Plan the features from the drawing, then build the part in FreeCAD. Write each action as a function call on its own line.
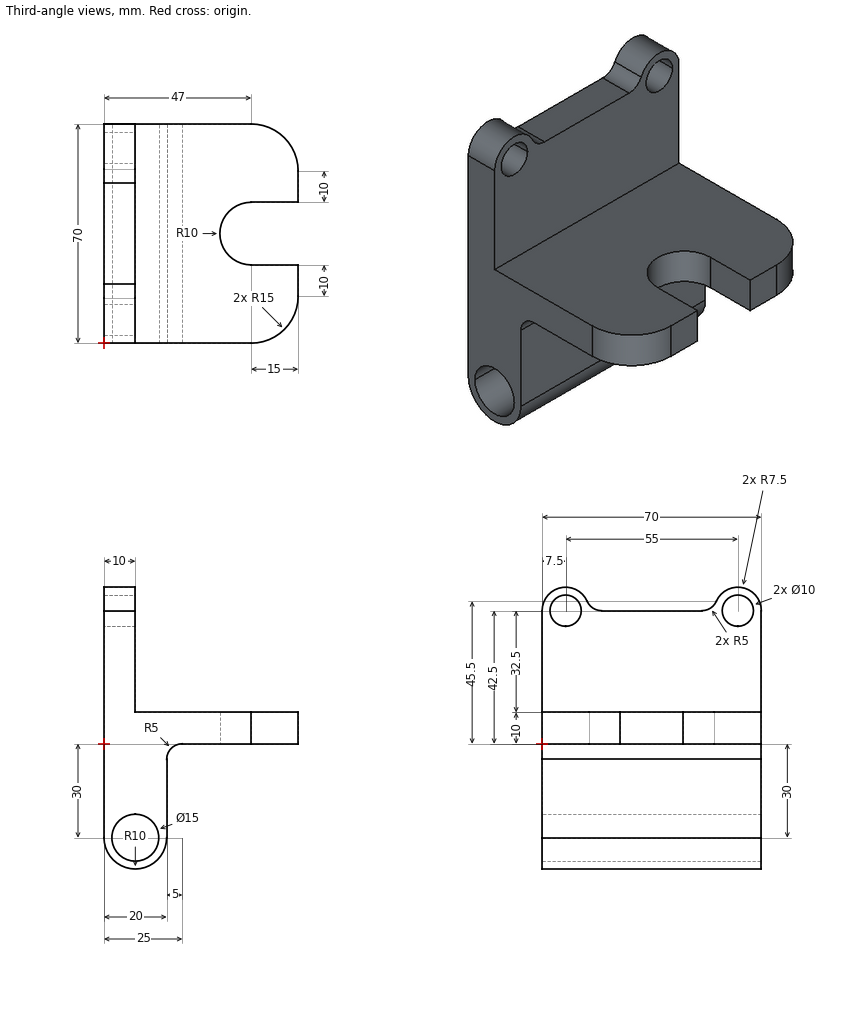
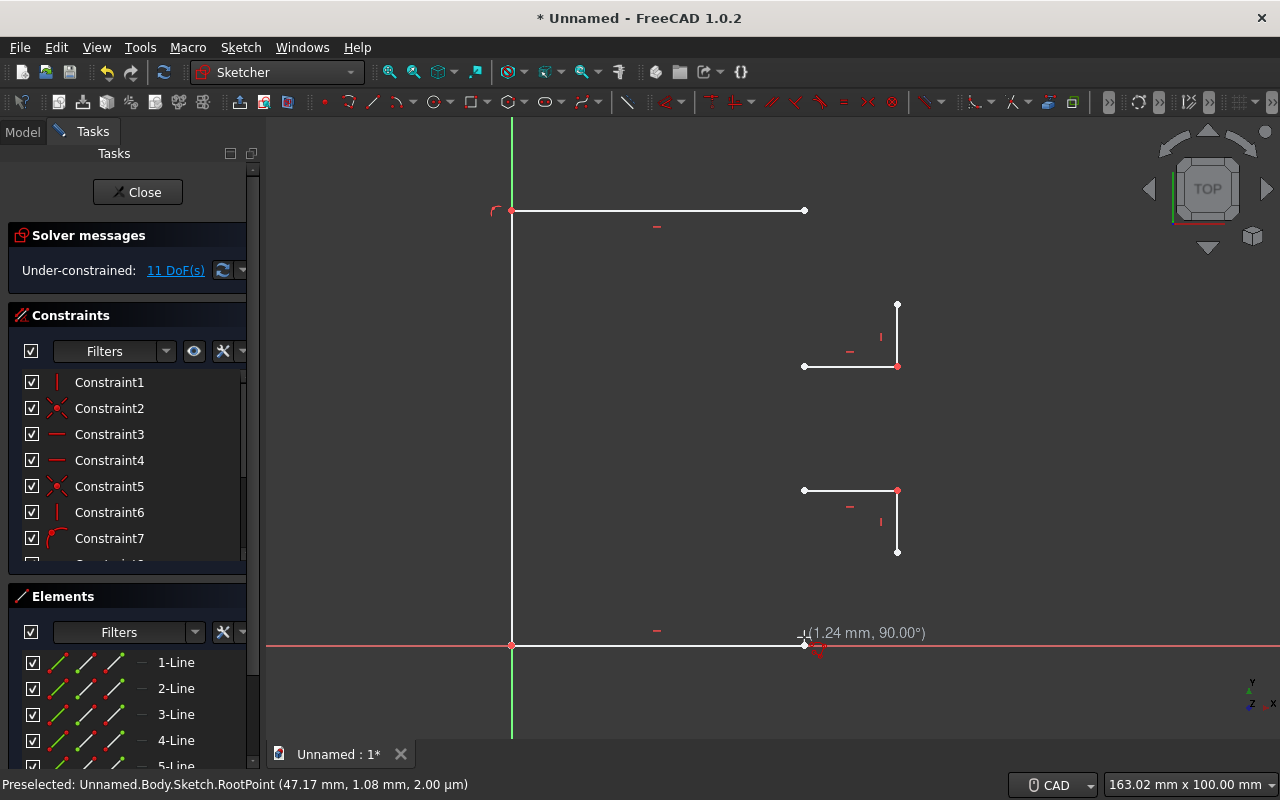
key(g)
key(3)
key(a)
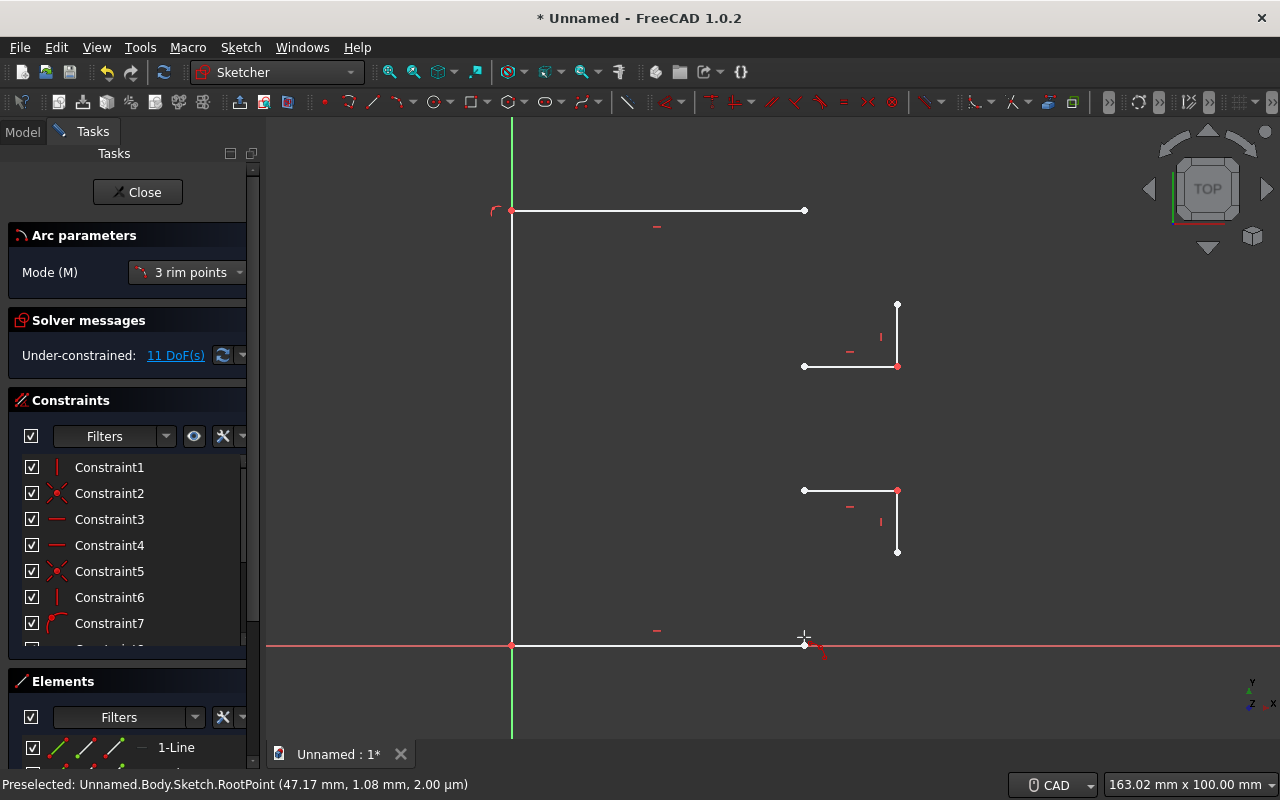
click(804, 491)
click(804, 367)
click(742, 428)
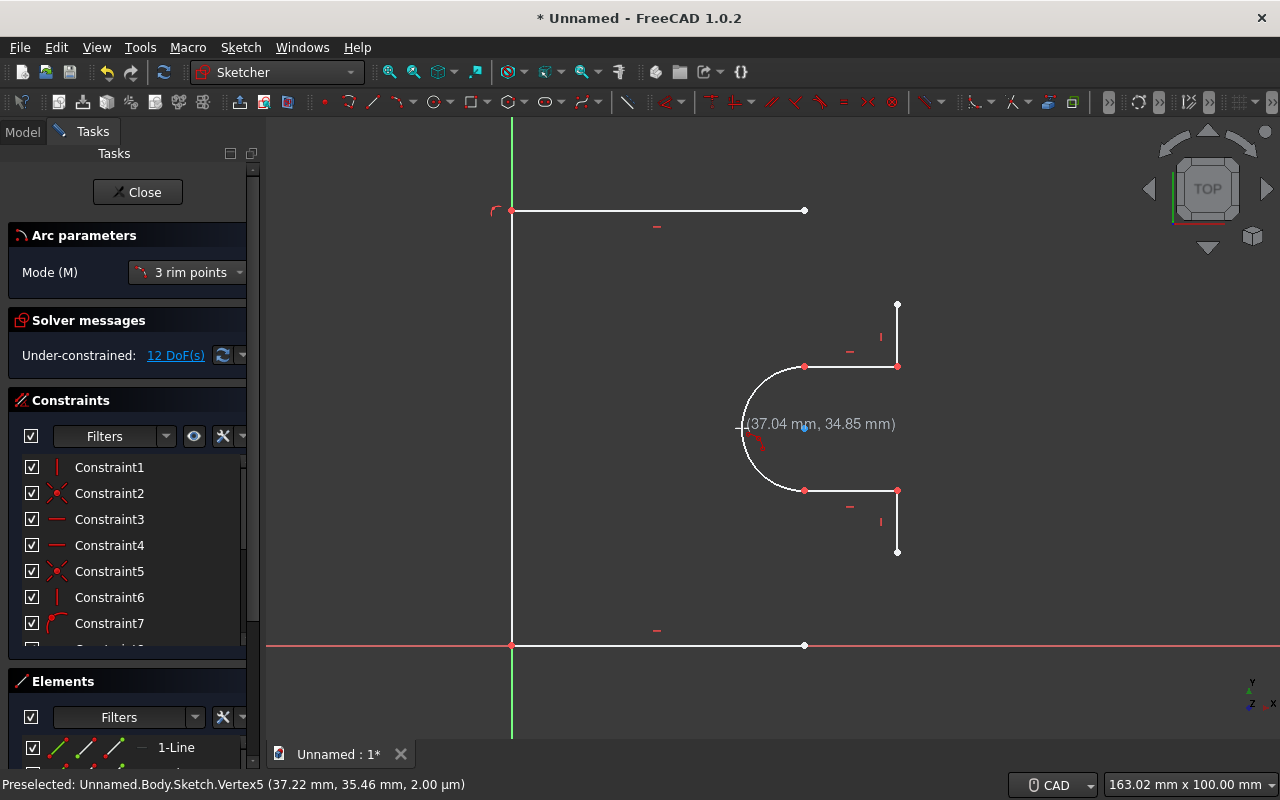
click(897, 305)
click(804, 211)
click(870, 238)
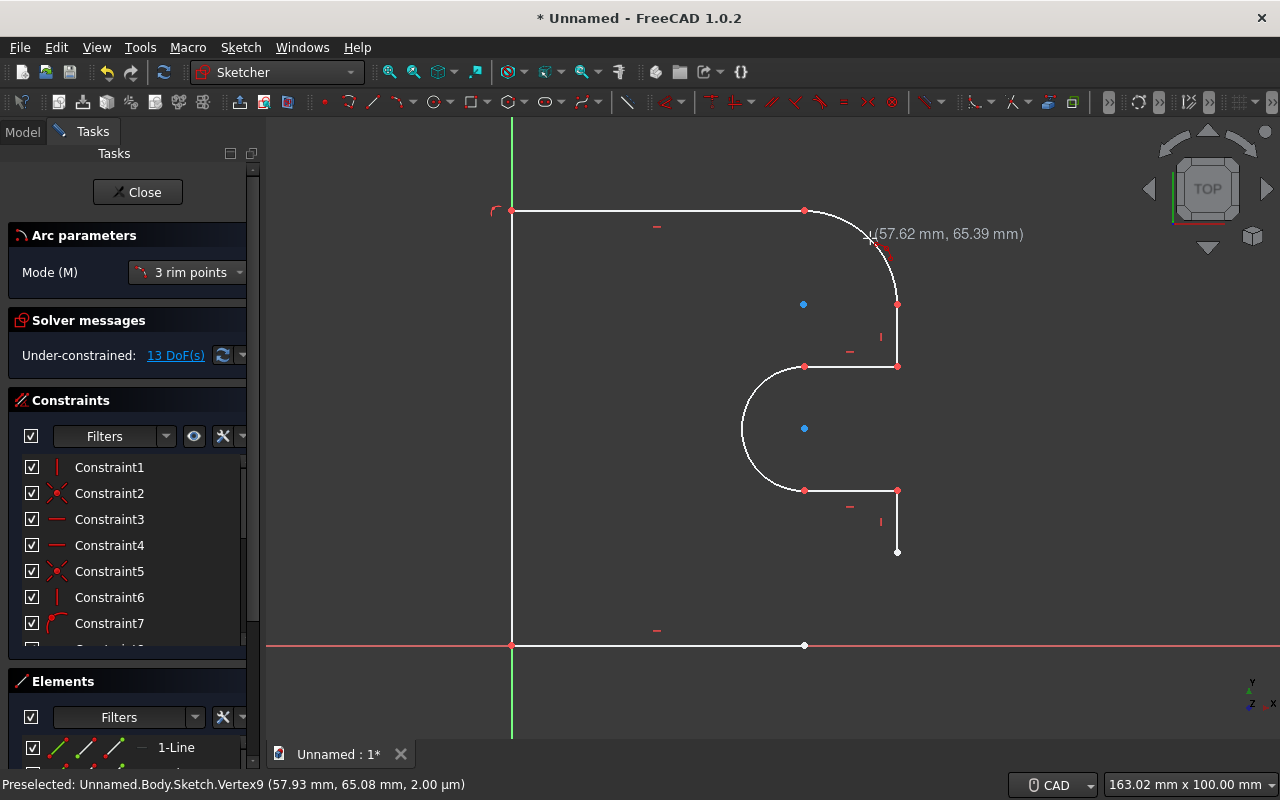
click(804, 646)
click(897, 553)
click(870, 618)
key(Escape)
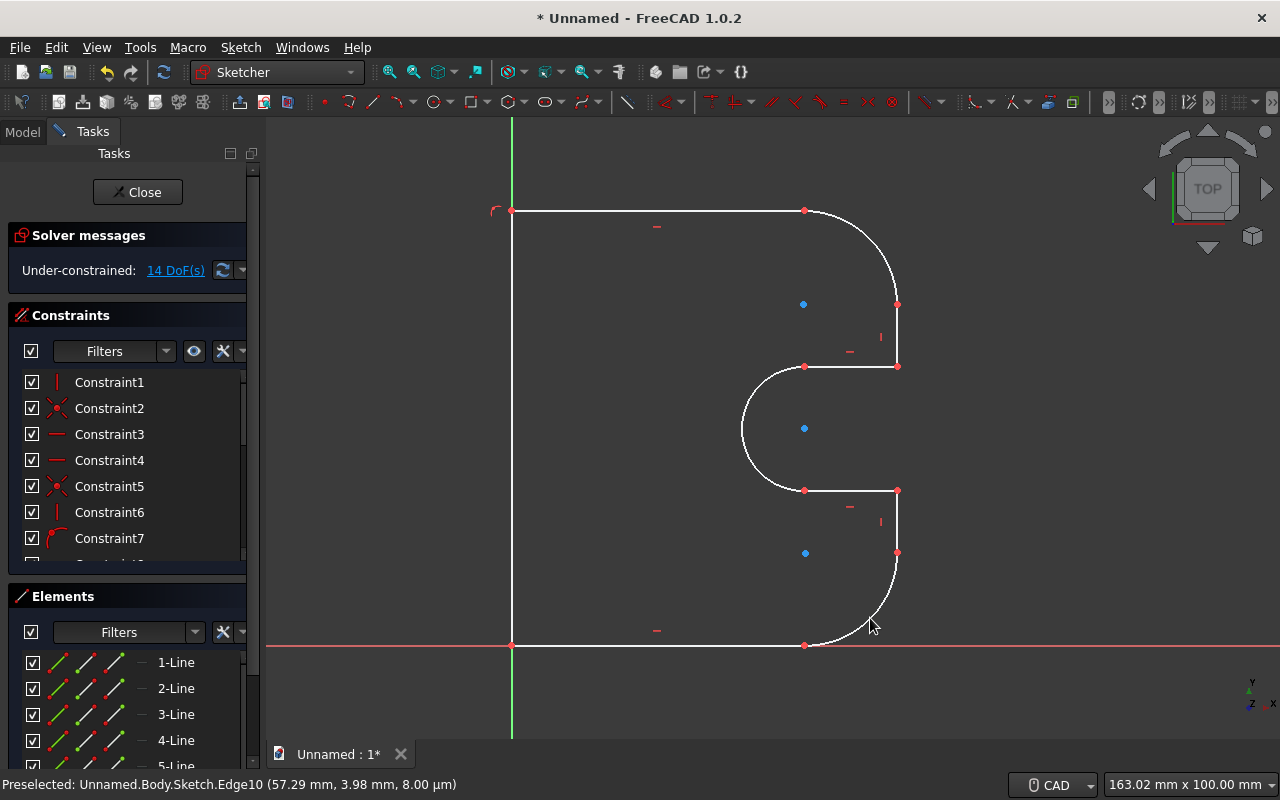
click(897, 534)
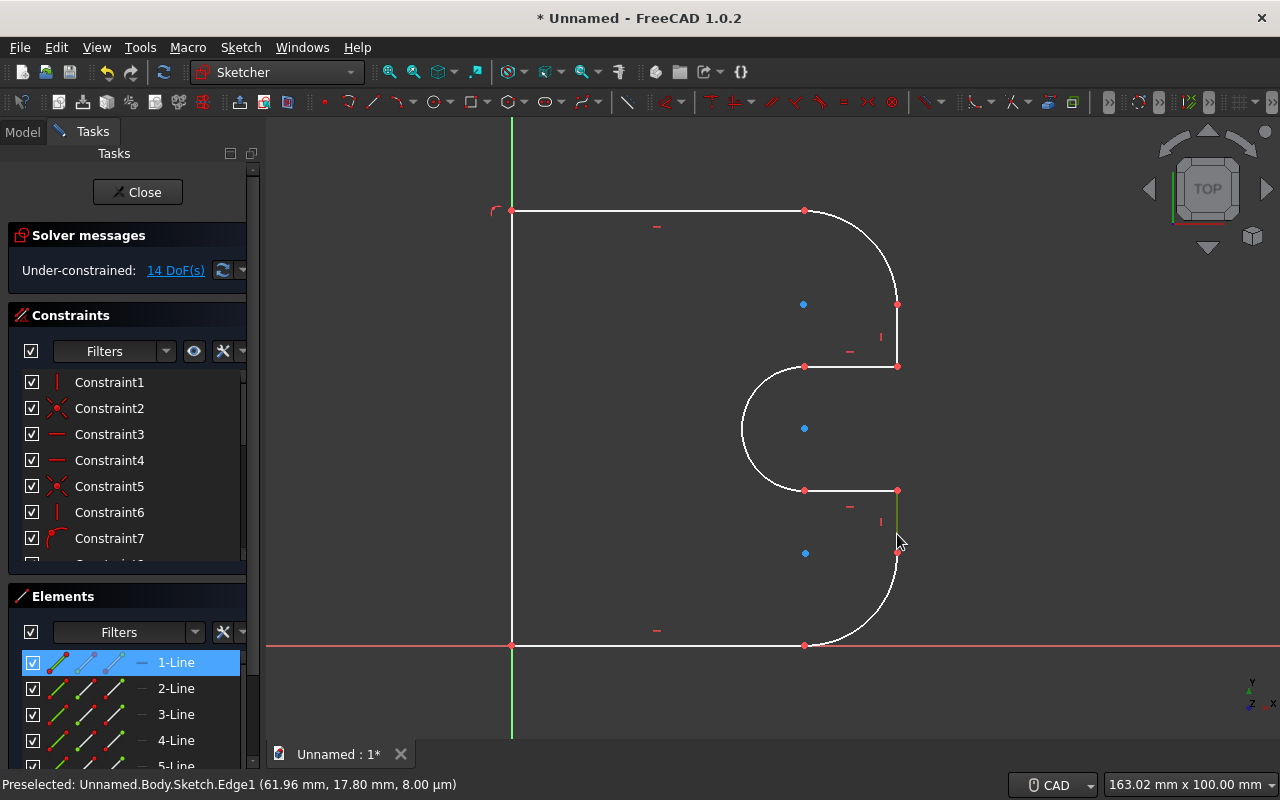
scroll(846, 636, up, 2)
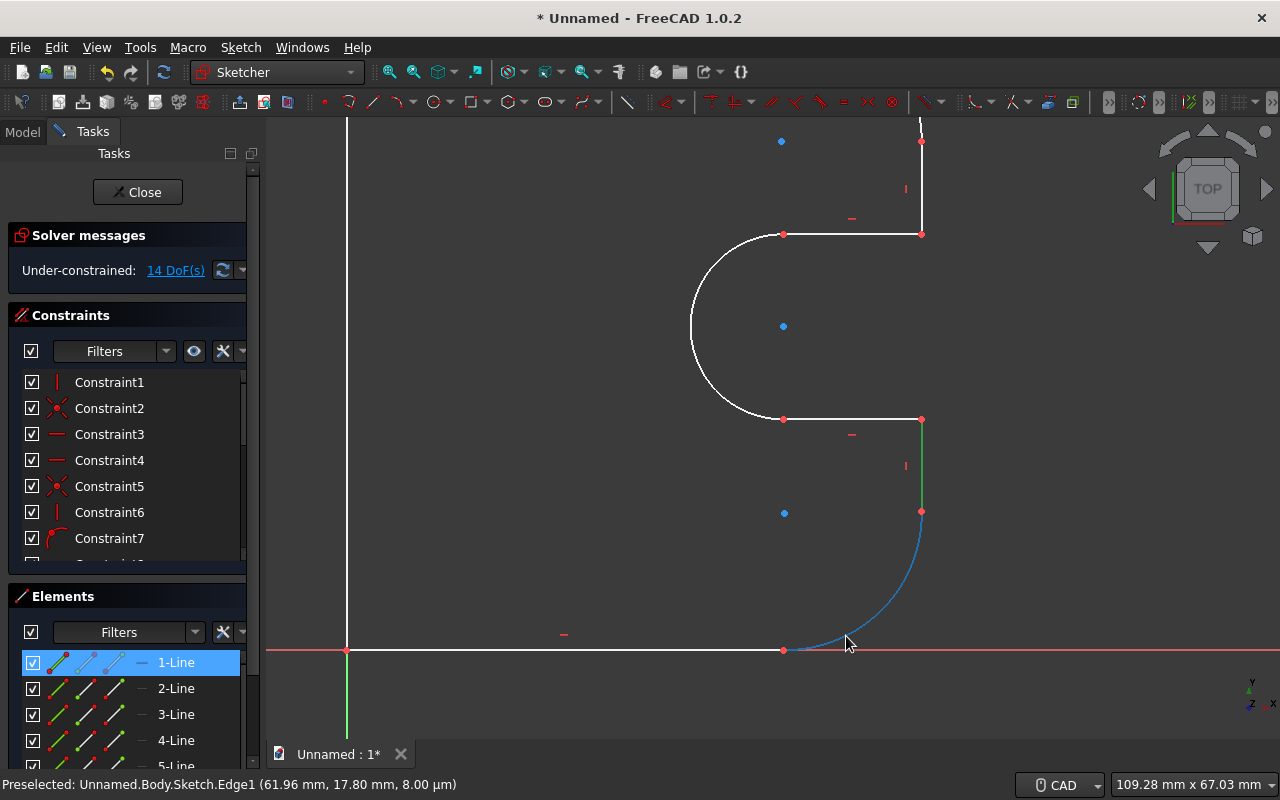
click(846, 636)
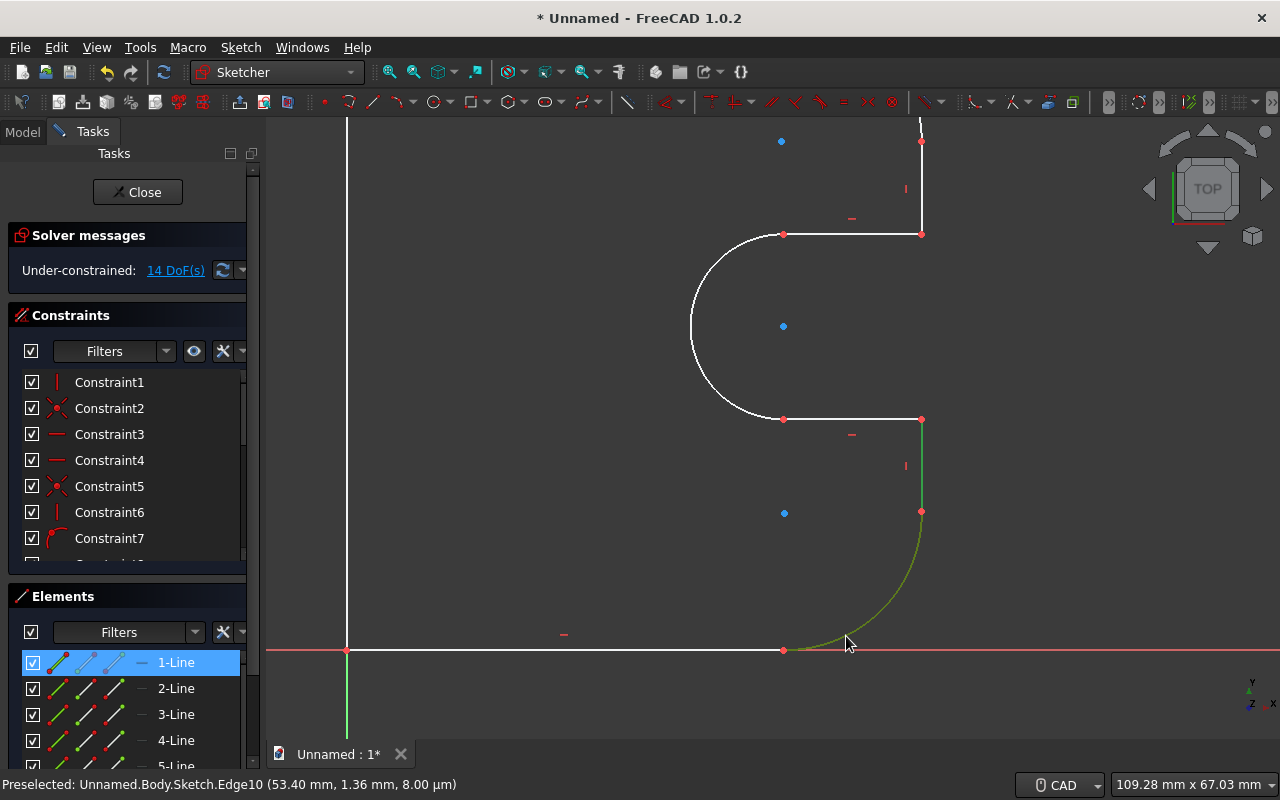
click(820, 102)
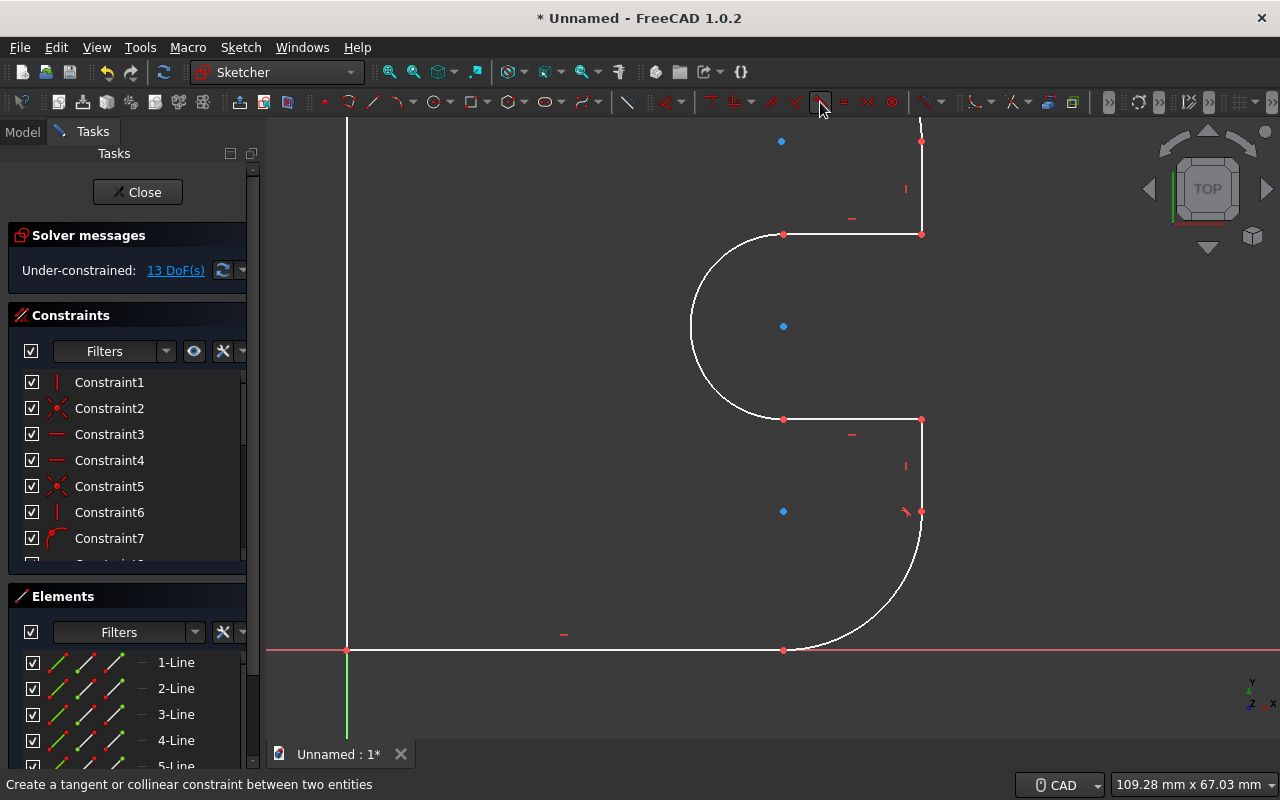
click(880, 419)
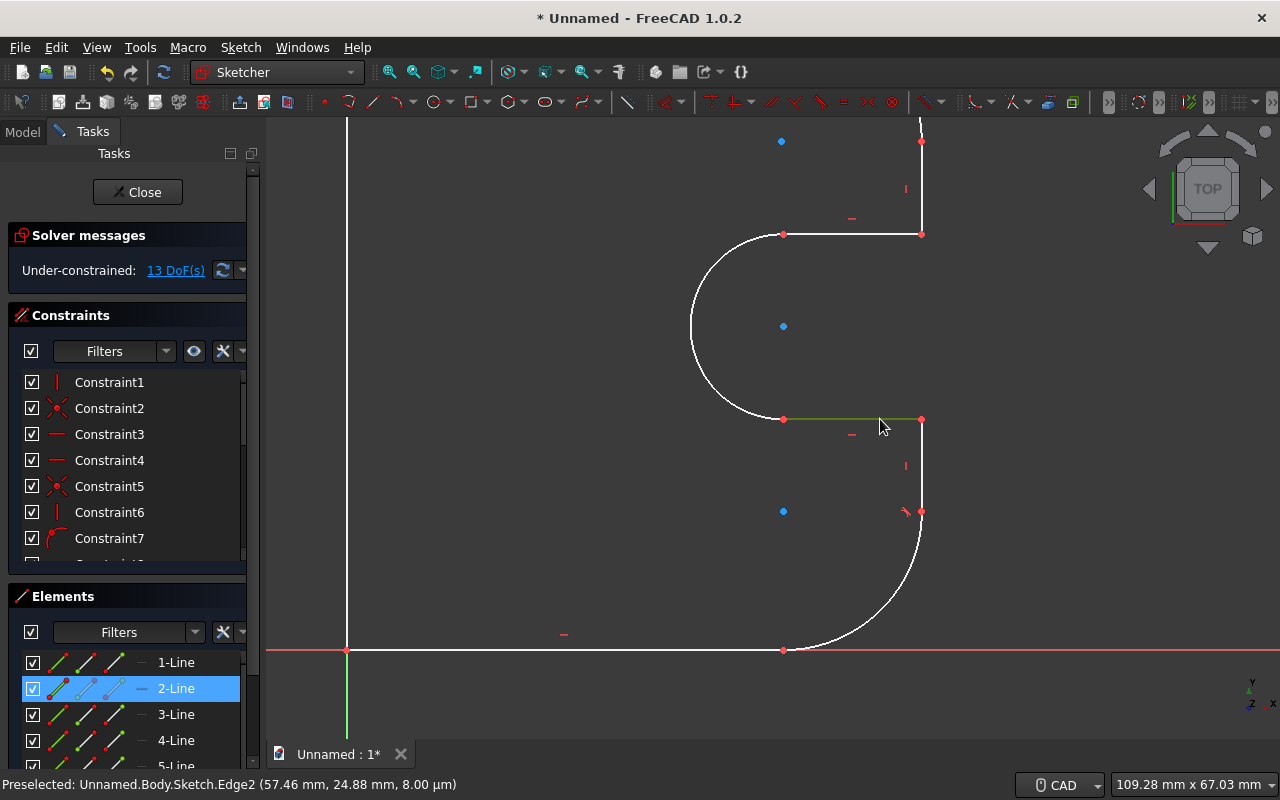
click(708, 272)